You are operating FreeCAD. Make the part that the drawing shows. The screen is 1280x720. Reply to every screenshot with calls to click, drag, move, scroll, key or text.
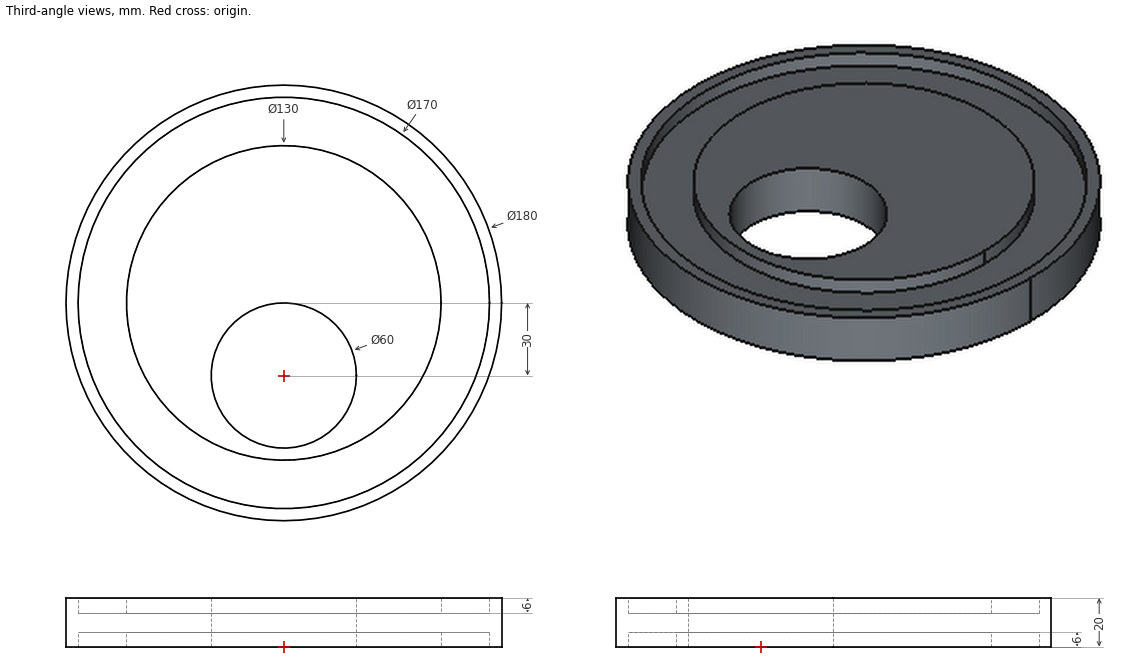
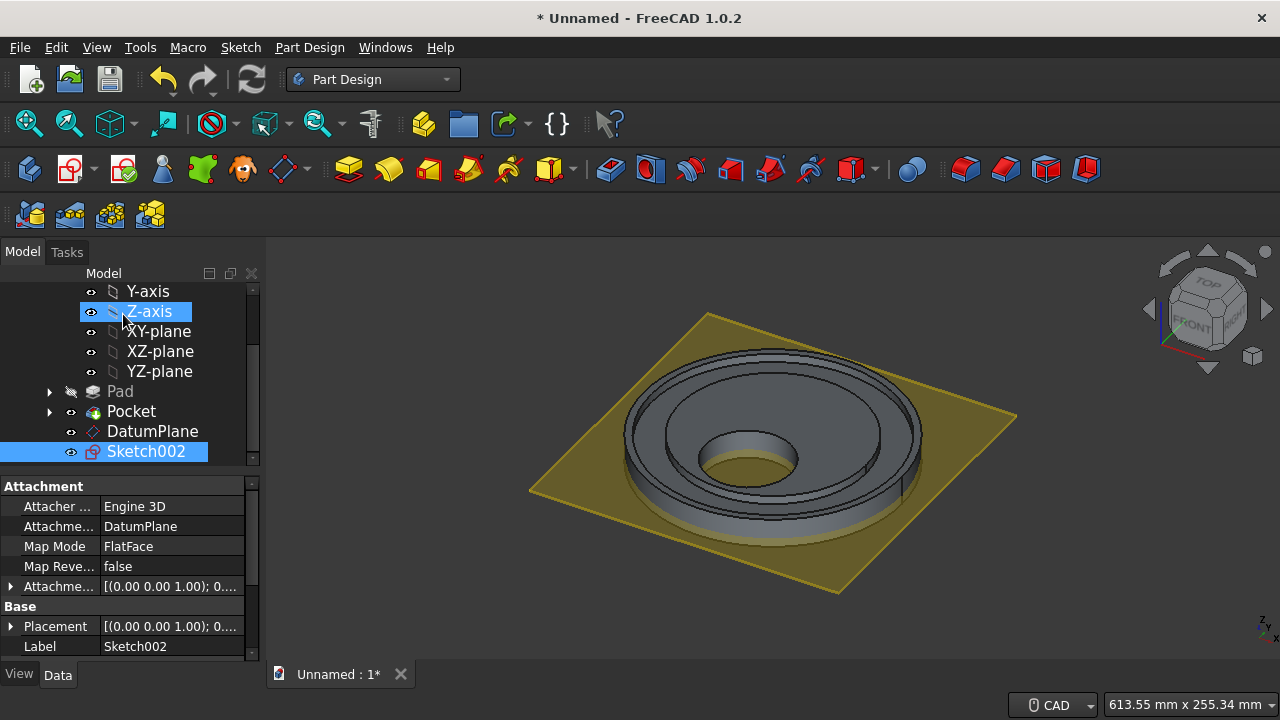
click(612, 170)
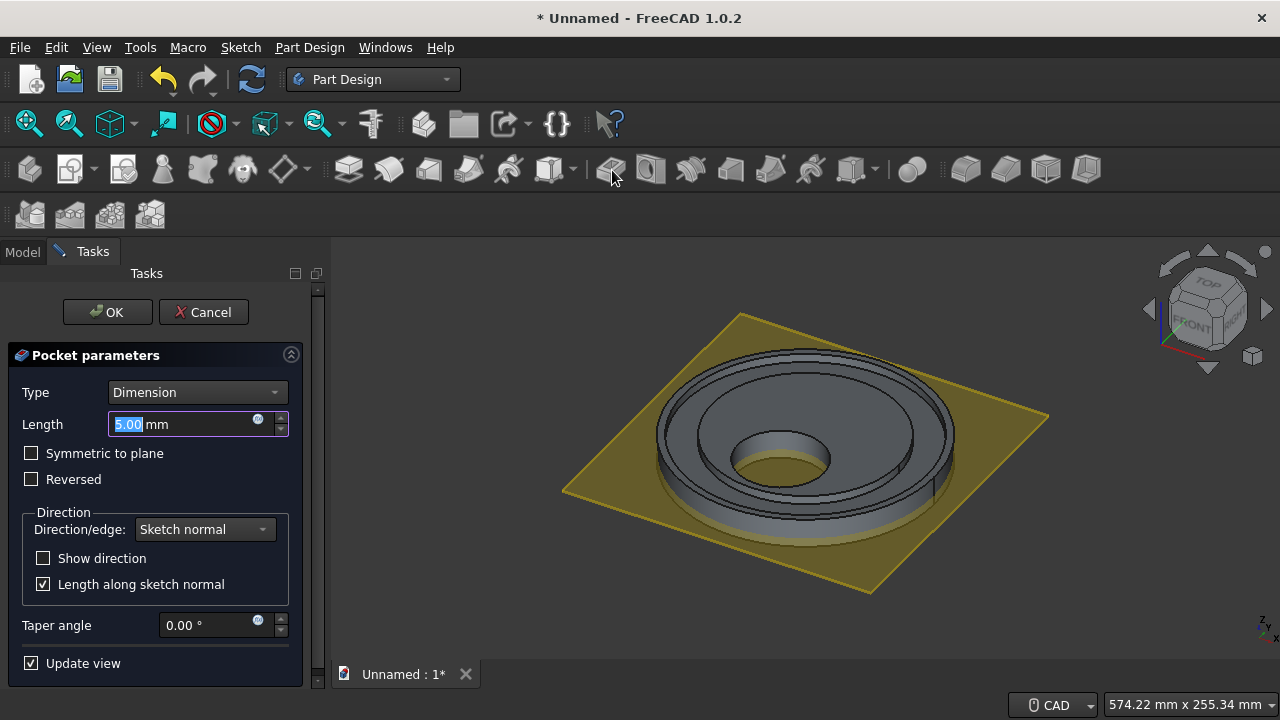
text(6)
key(Tab)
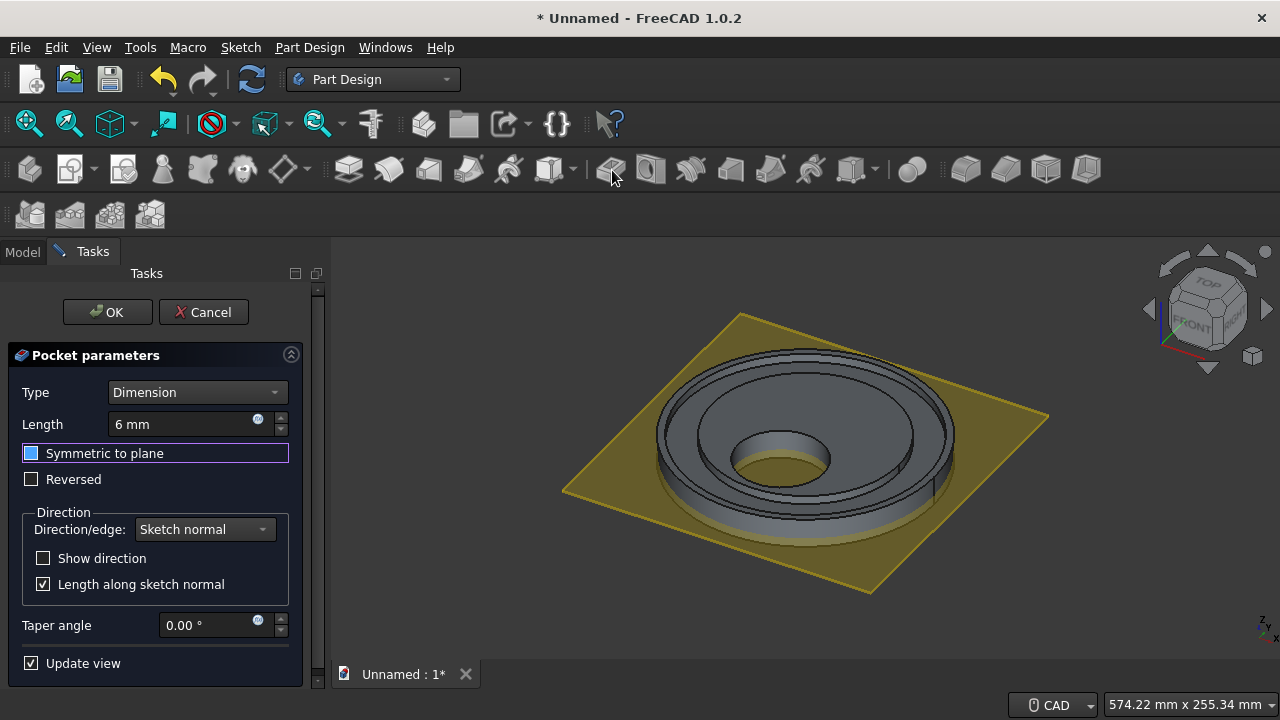
click(108, 312)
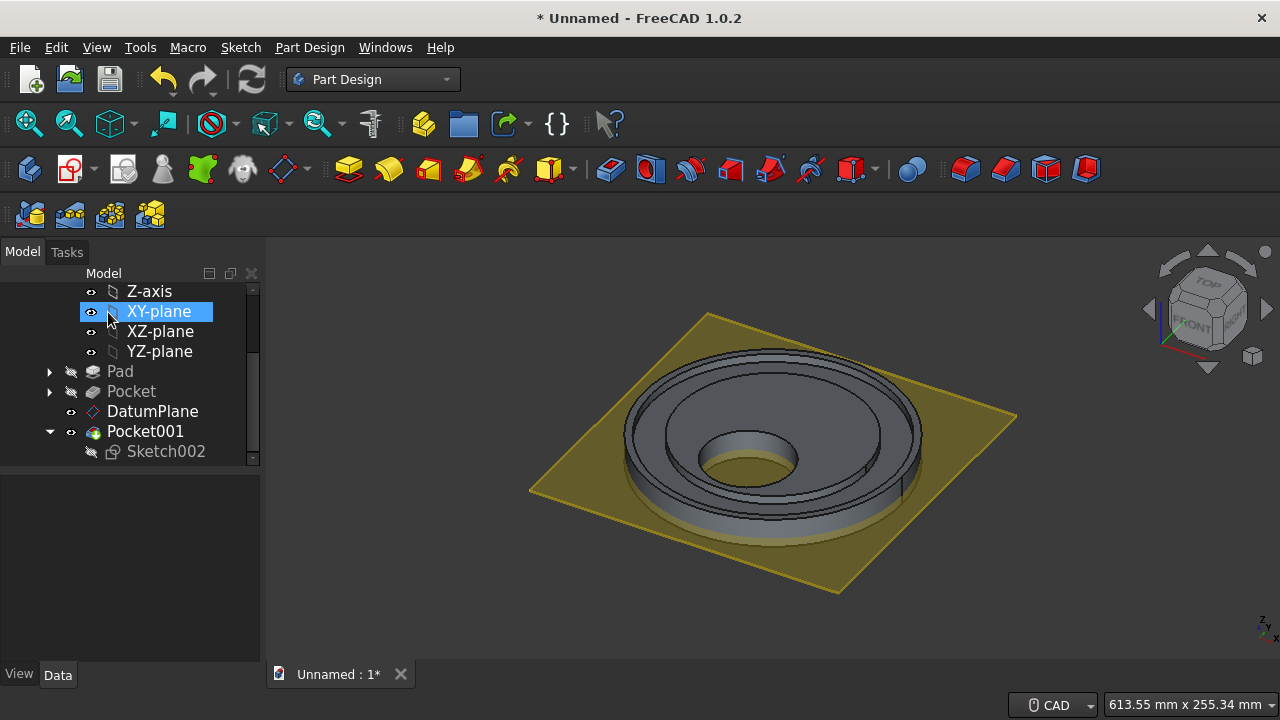
click(116, 412)
key(space)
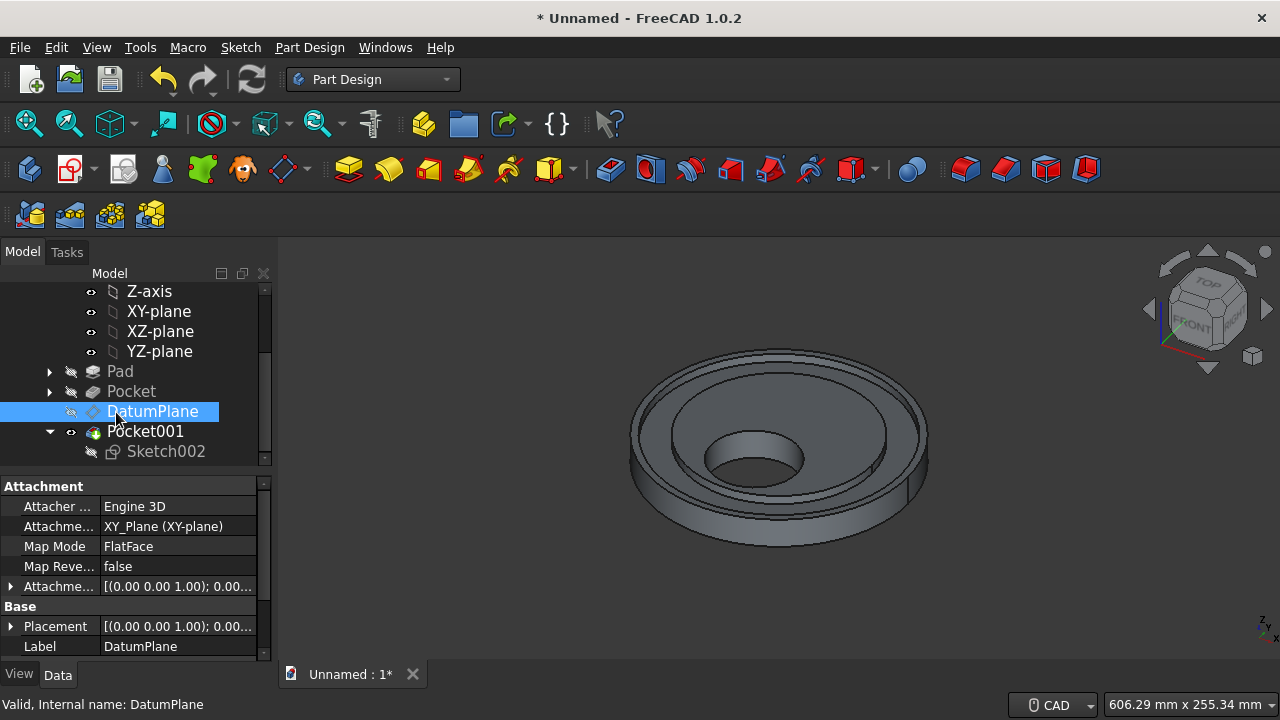
key(0)